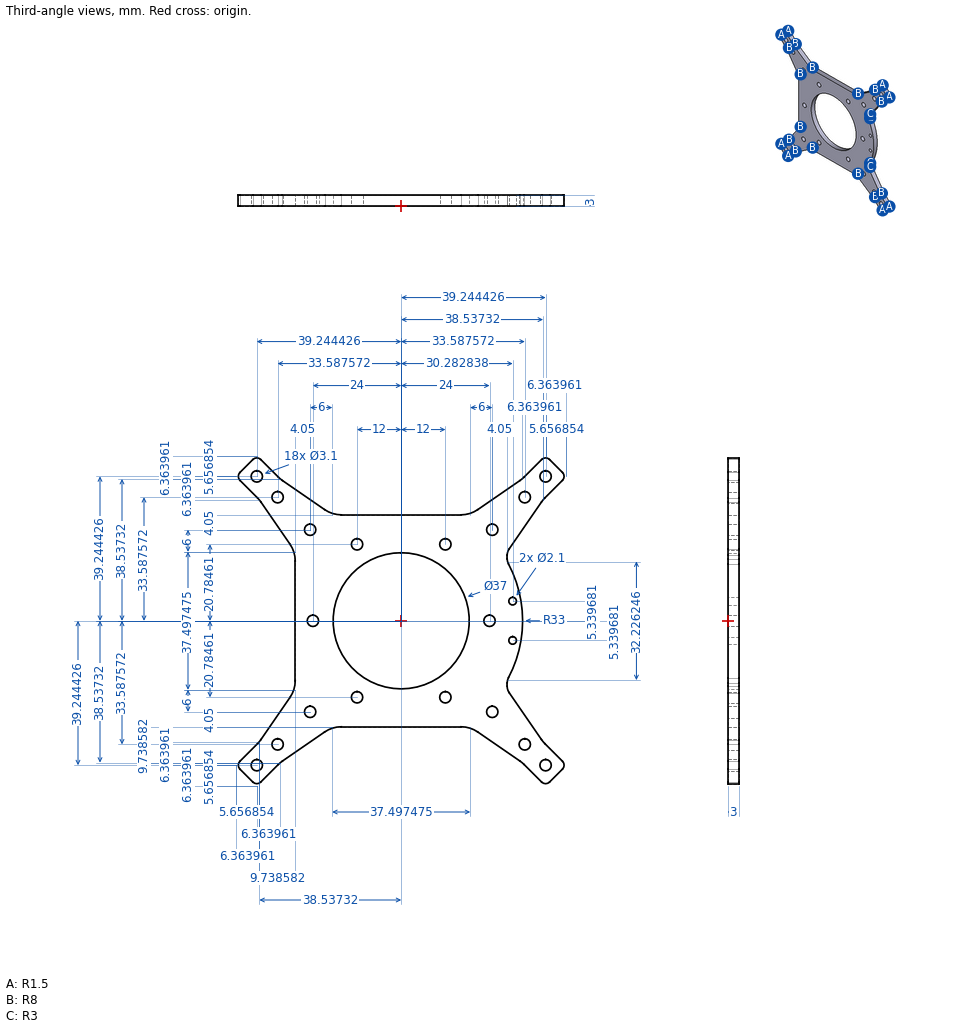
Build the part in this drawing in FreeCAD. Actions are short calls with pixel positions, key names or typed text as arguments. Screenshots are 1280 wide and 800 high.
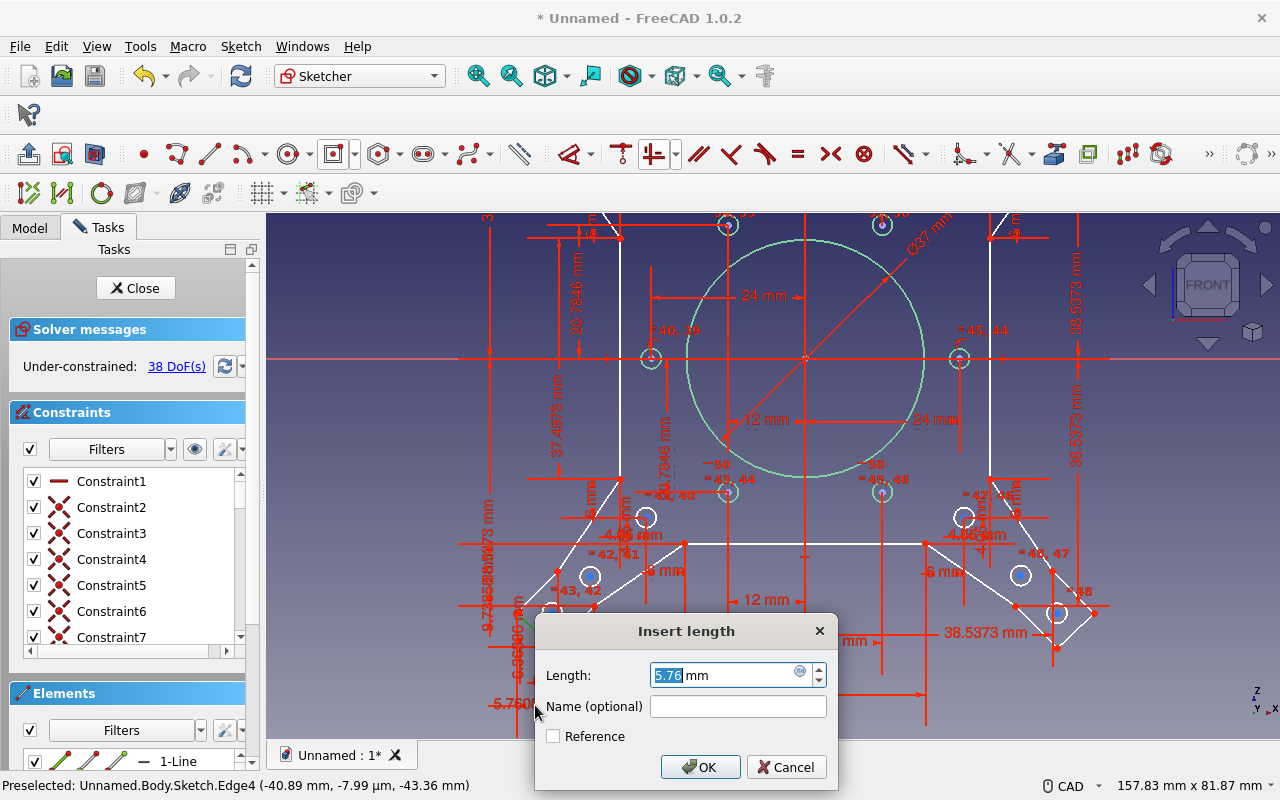
text(5.656854)
key(Return)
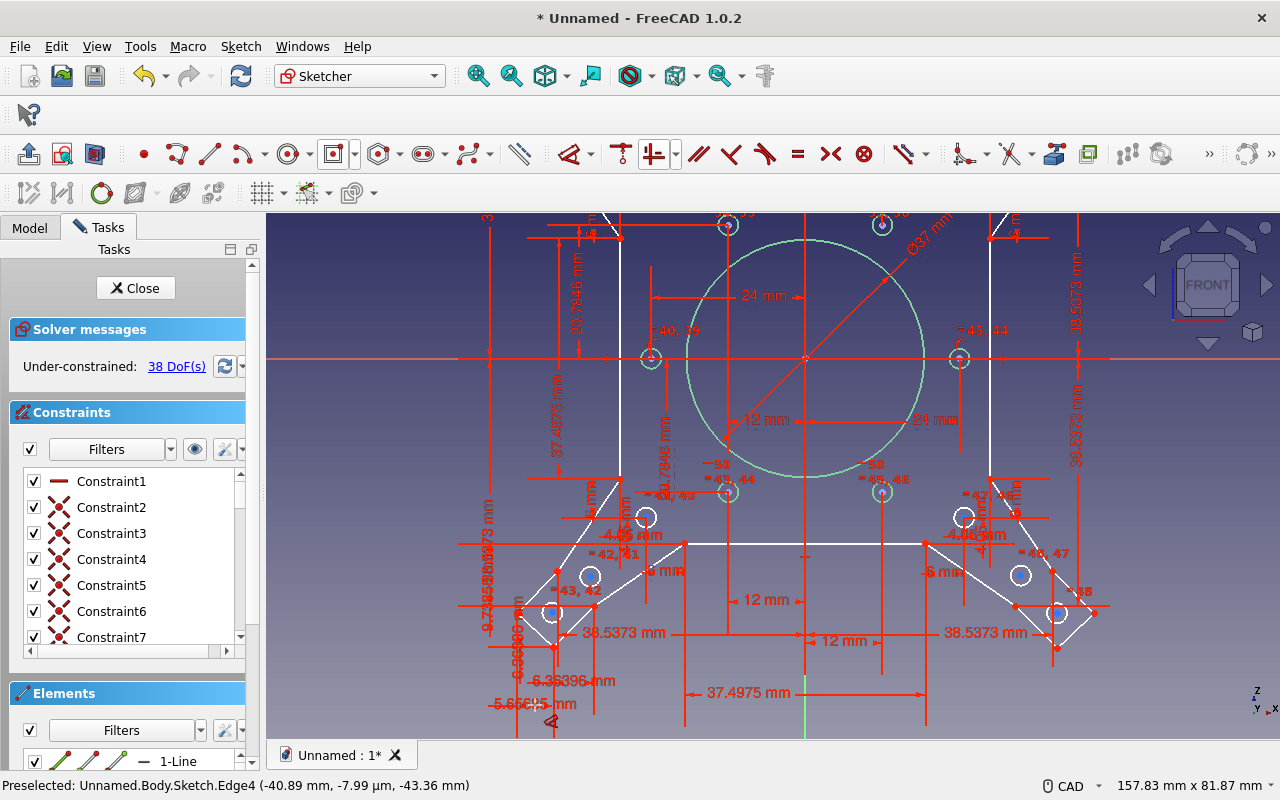
click(543, 637)
click(435, 630)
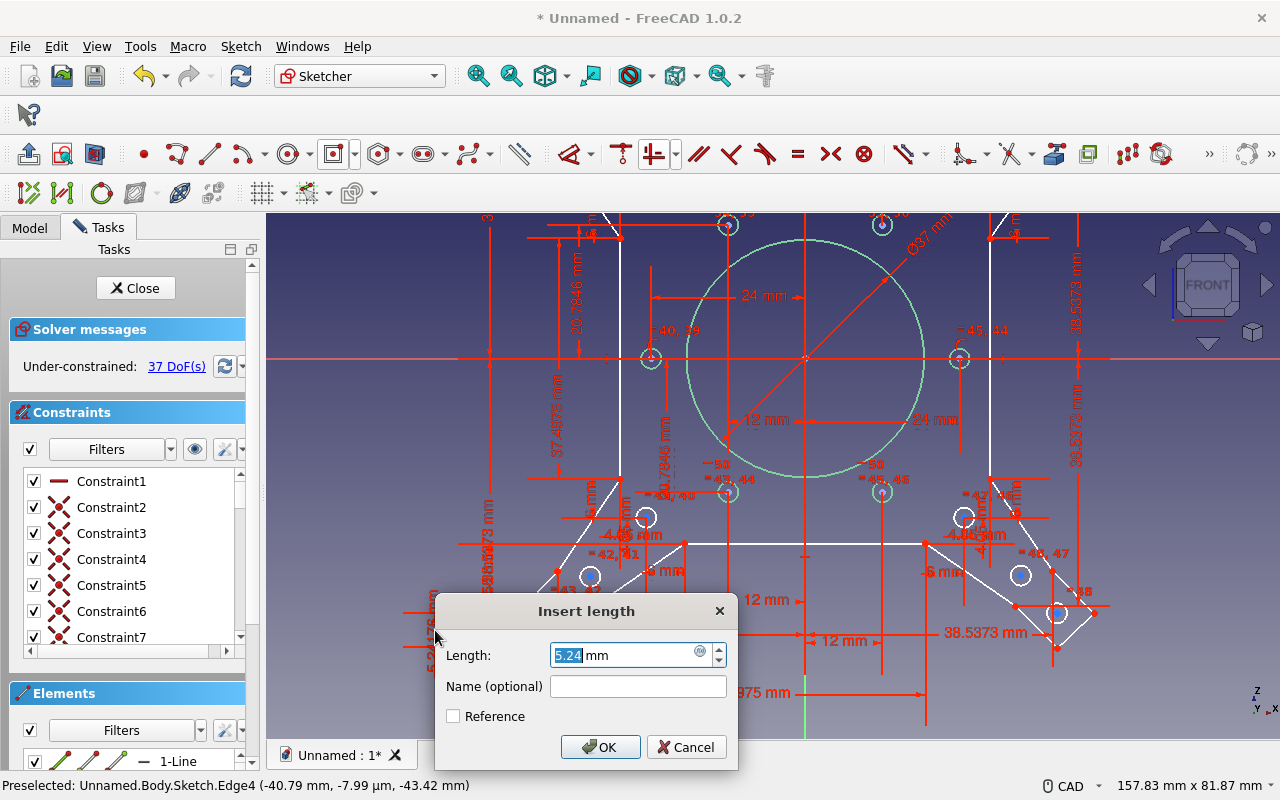
text(5.656854)
key(Return)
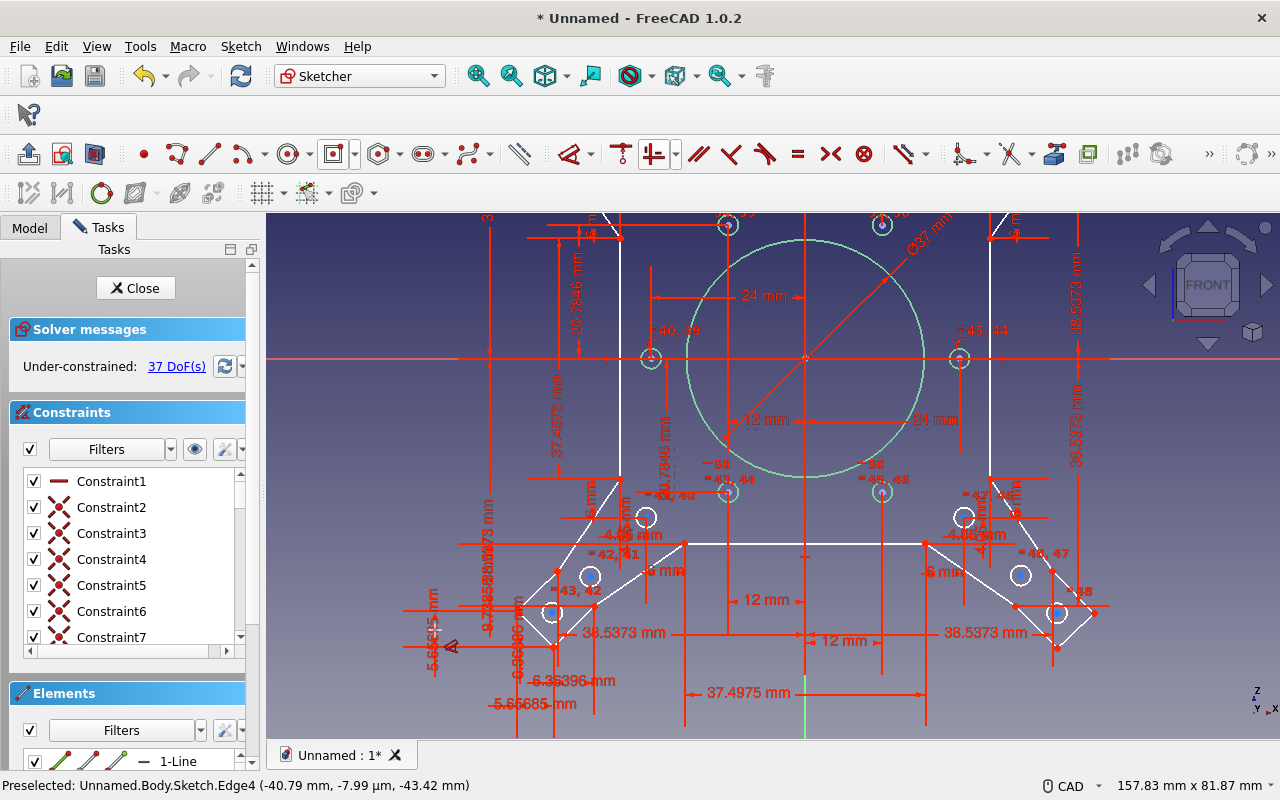
click(529, 599)
click(538, 466)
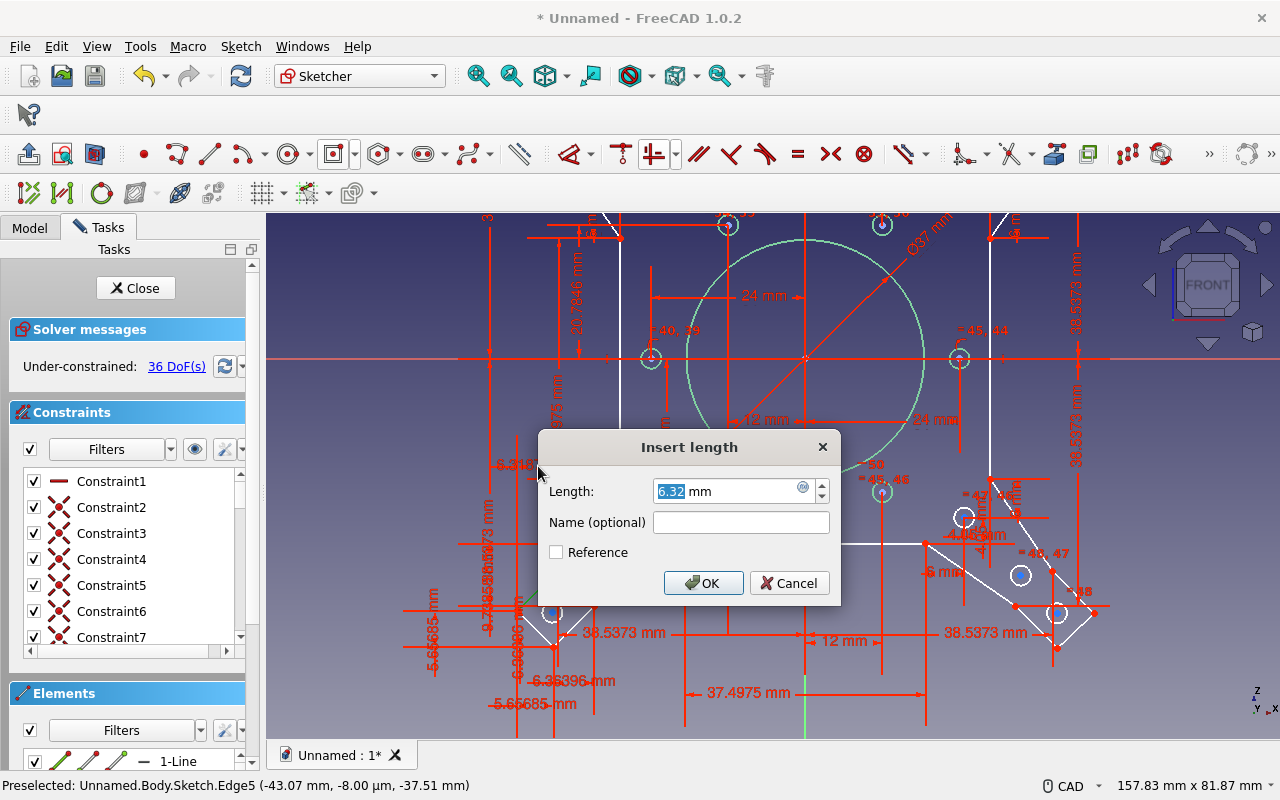
text(6.363961)
key(Return)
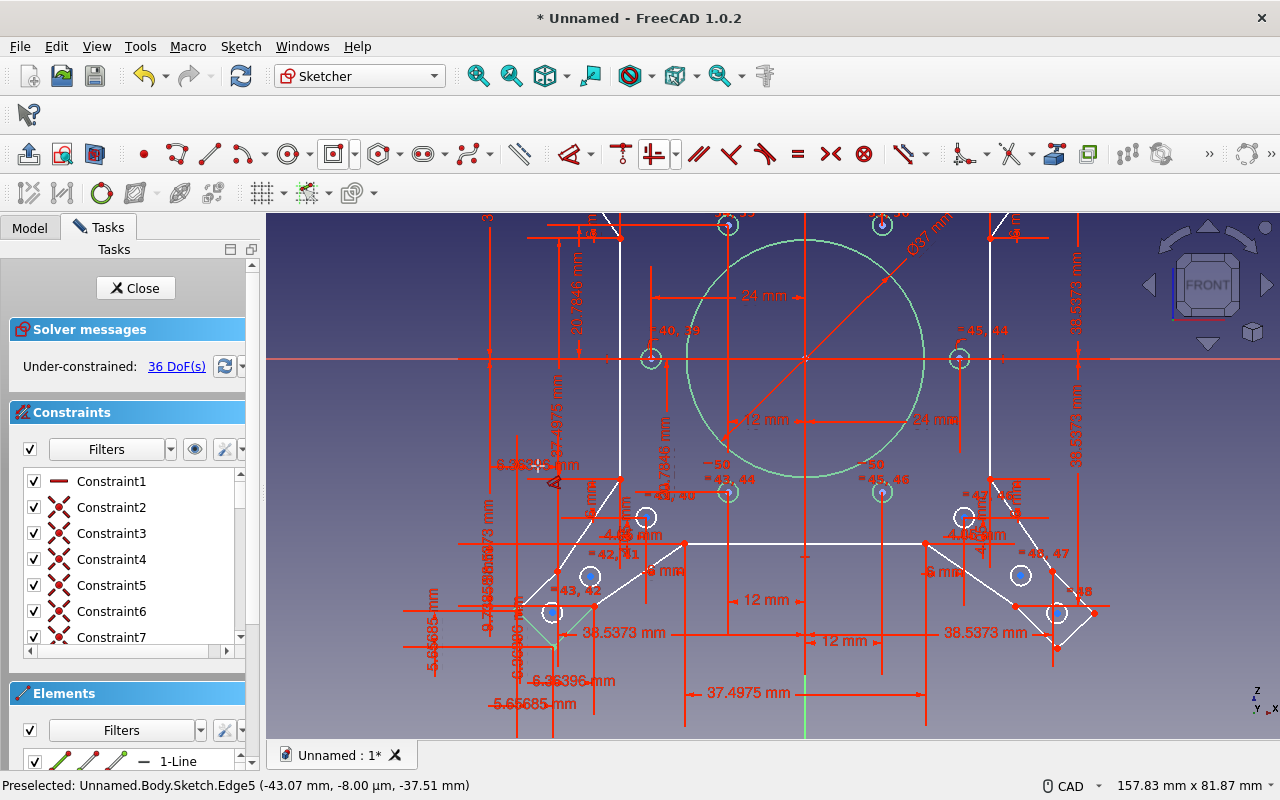
click(529, 599)
click(640, 600)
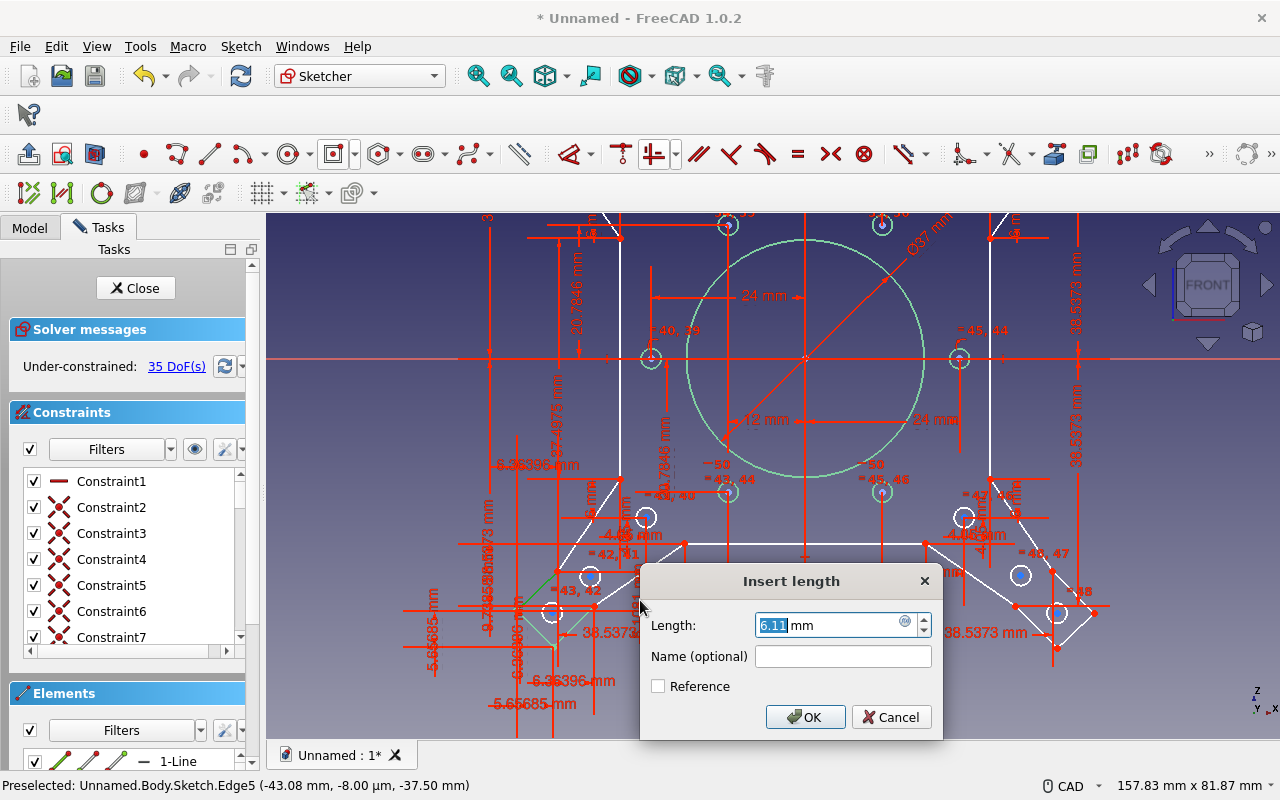
text(6.363961)
key(Return)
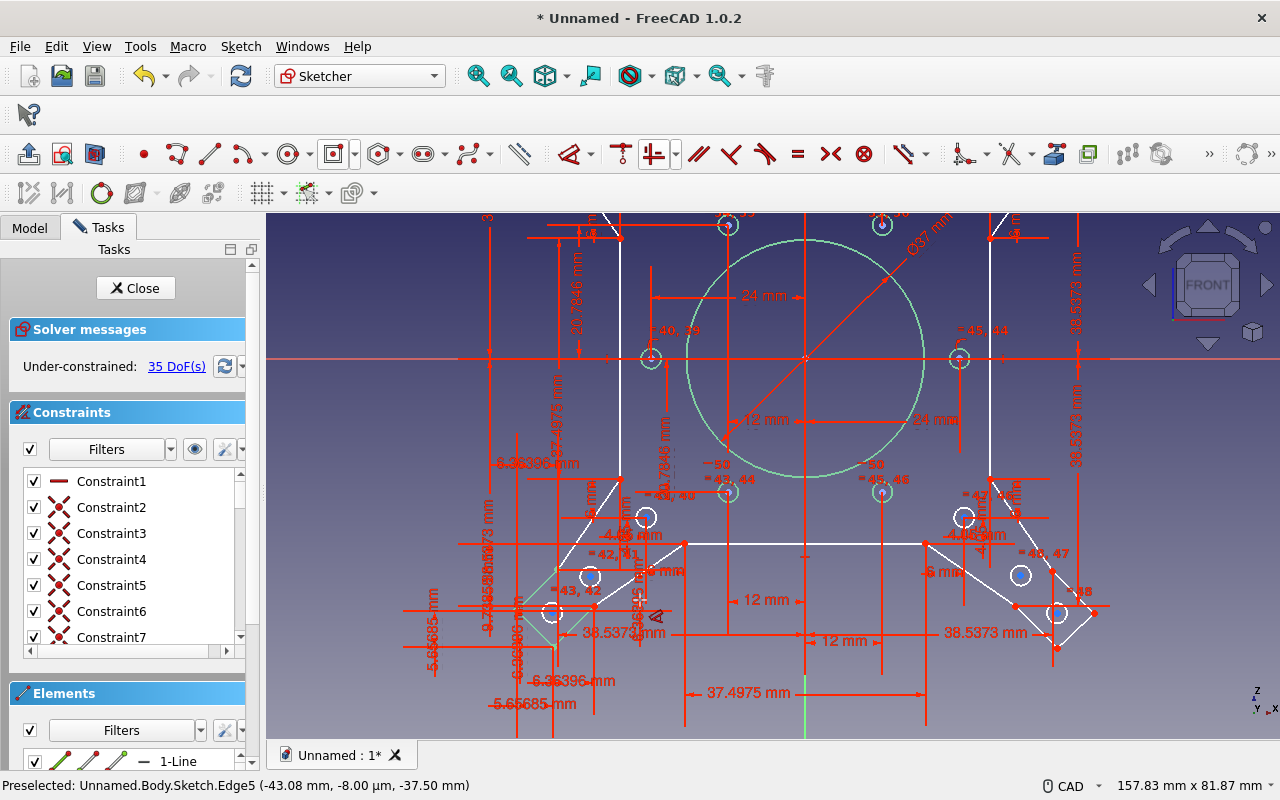
click(577, 543)
click(589, 445)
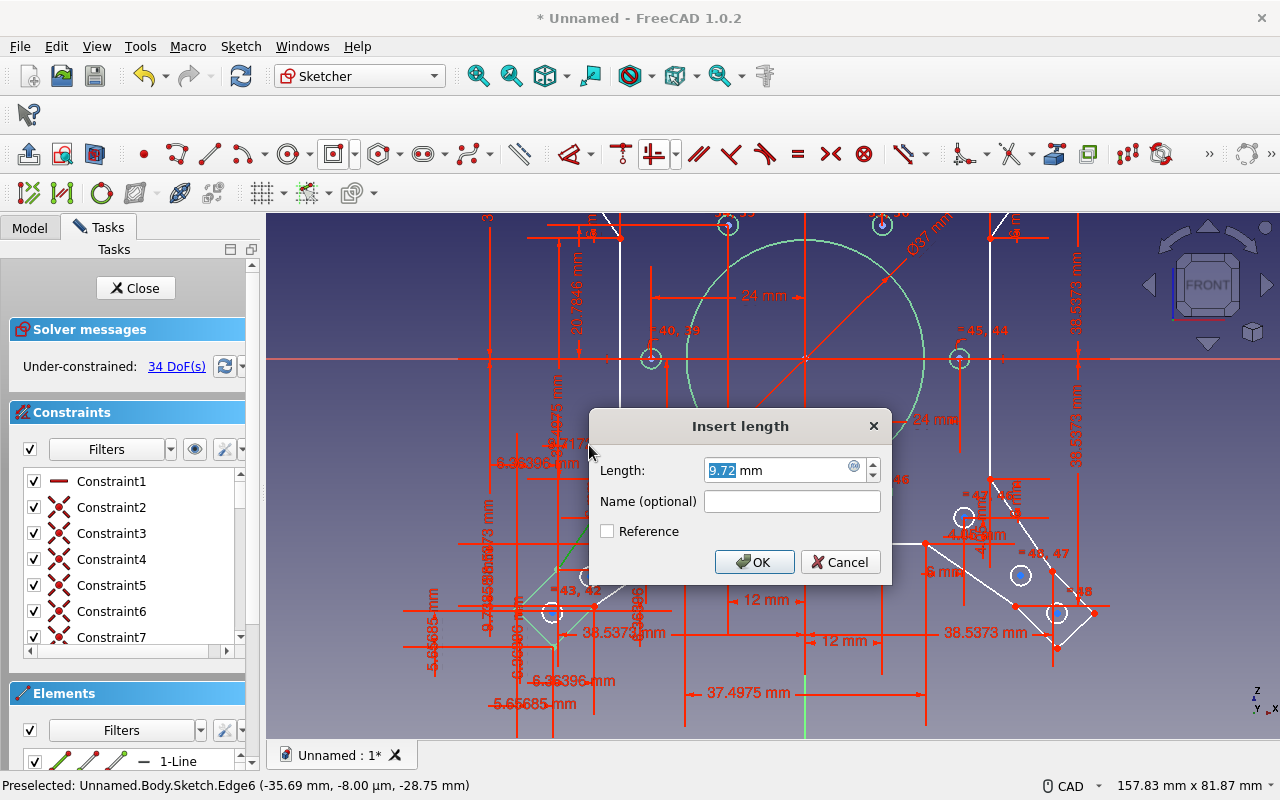
text(9.738582)
key(Return)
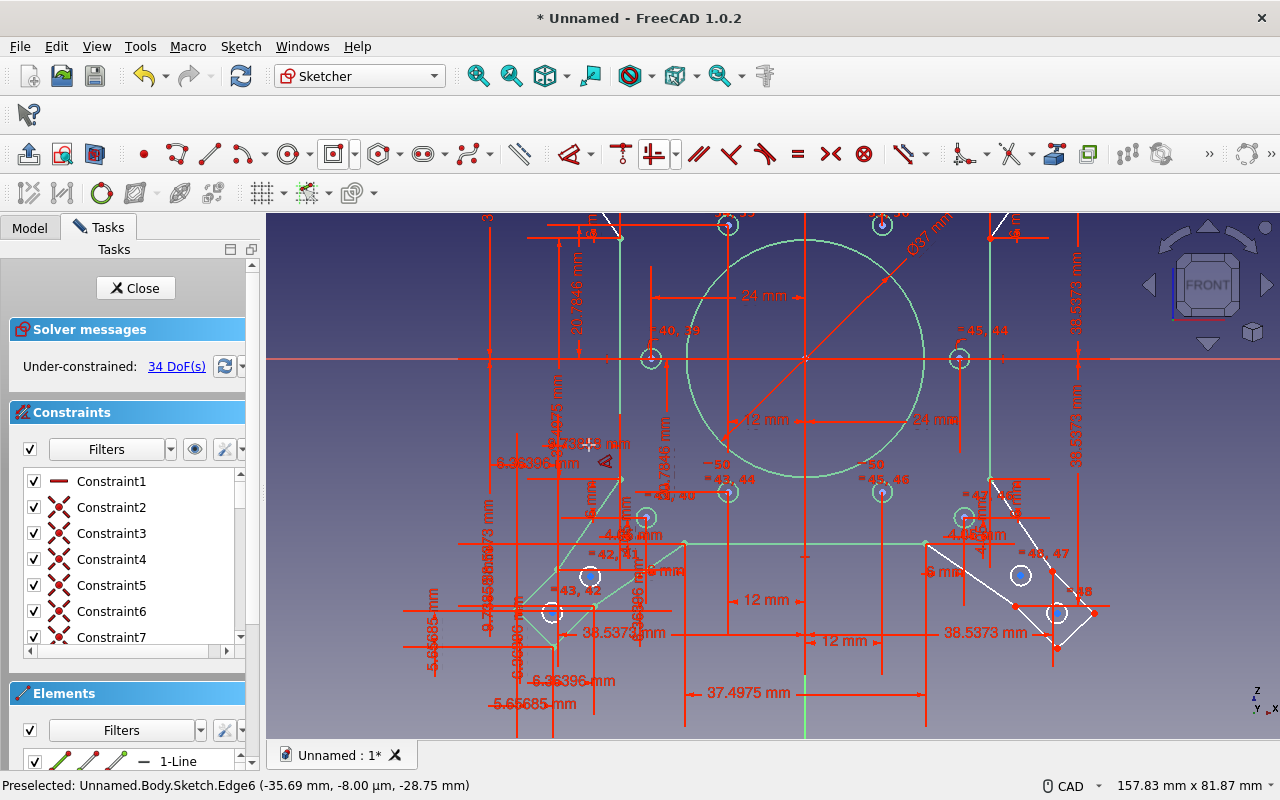
scroll(582, 619, down, 3)